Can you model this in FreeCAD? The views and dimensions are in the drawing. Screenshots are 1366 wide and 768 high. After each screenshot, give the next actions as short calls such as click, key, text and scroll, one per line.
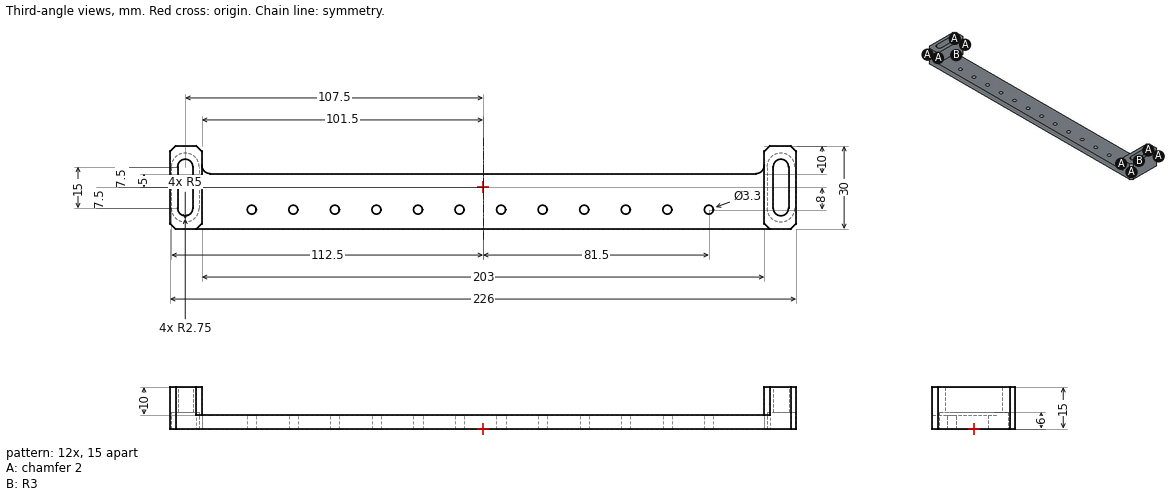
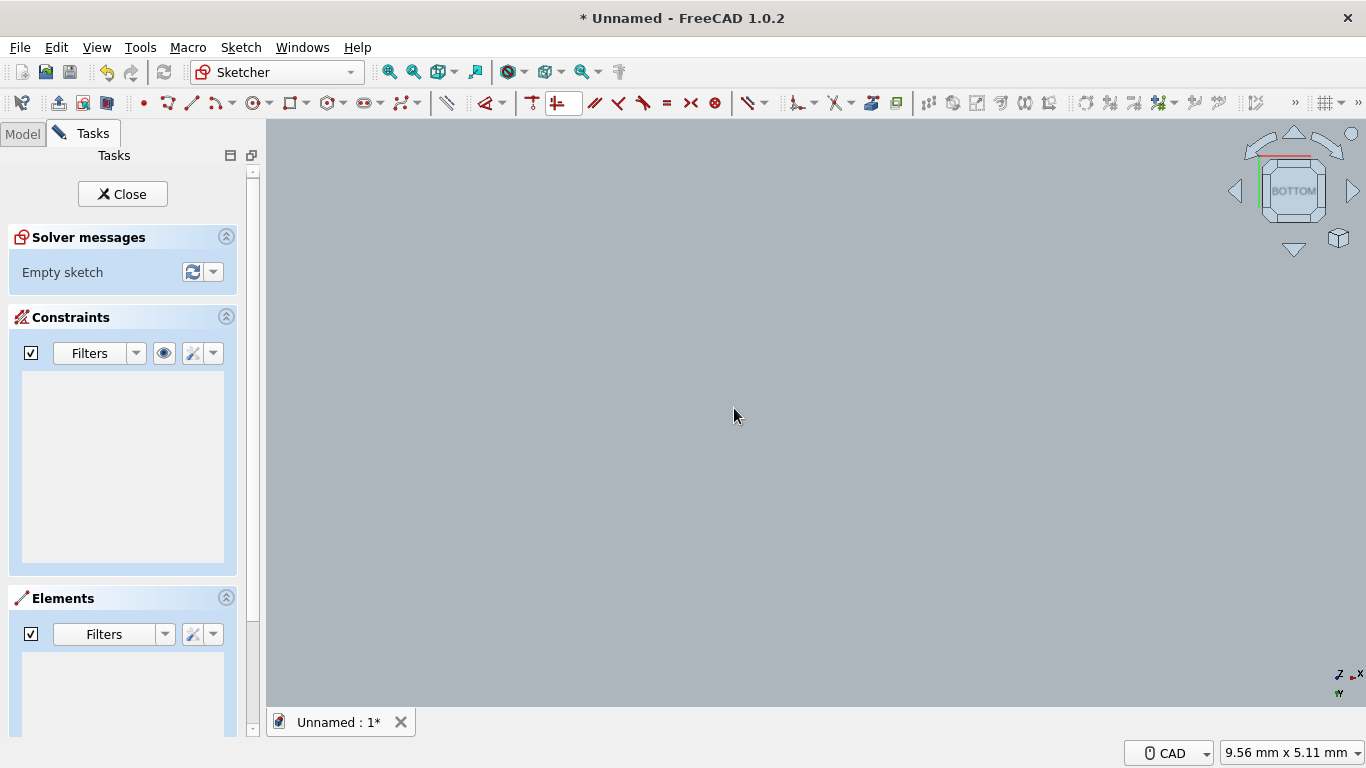
click(254, 104)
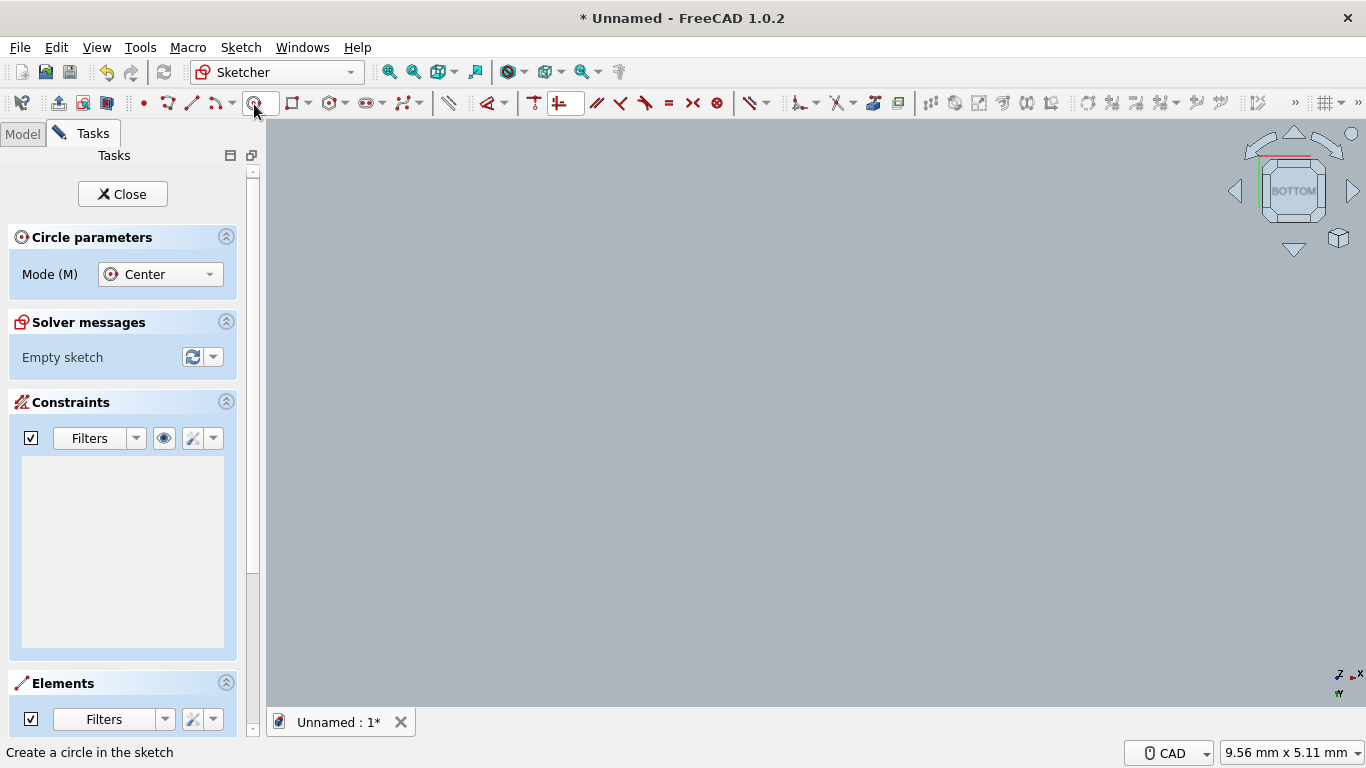
click(747, 413)
move(882, 279)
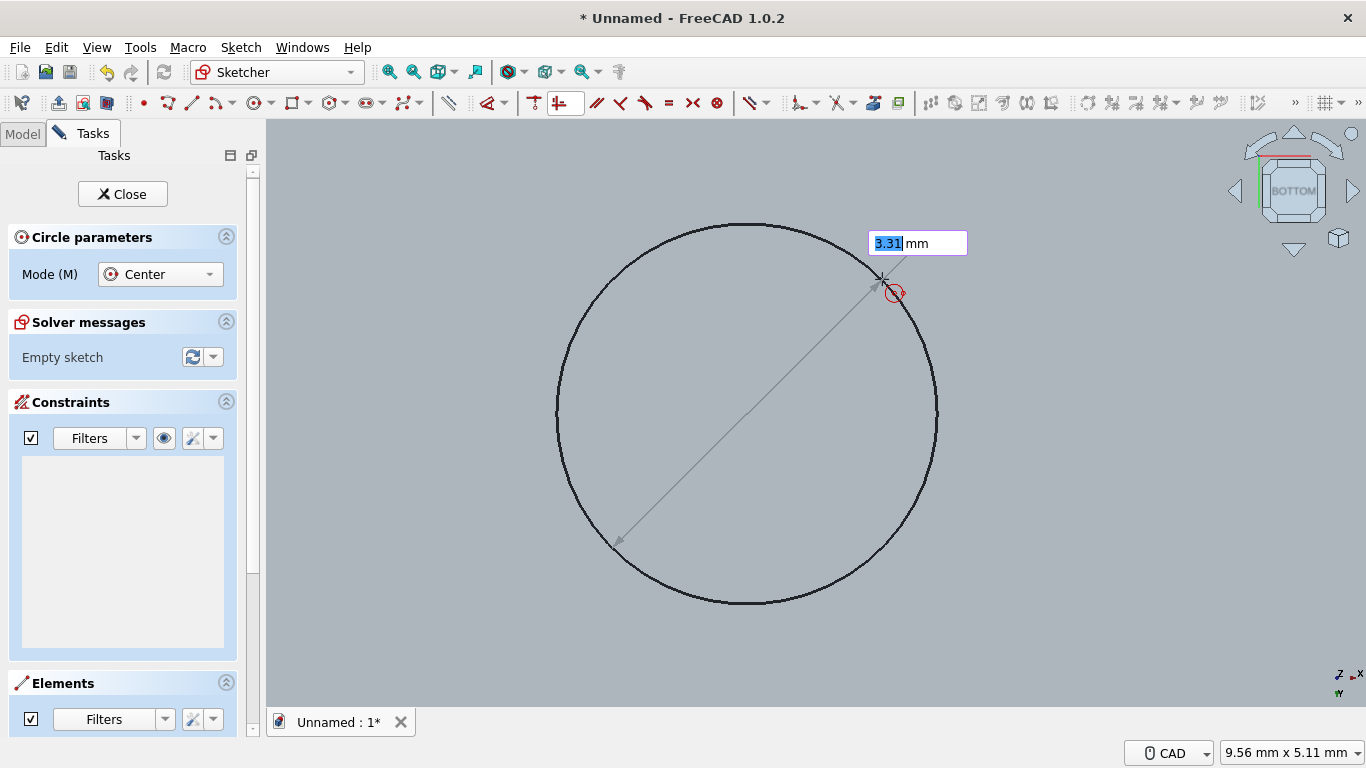
text(3.3)
key(Return)
key(Escape)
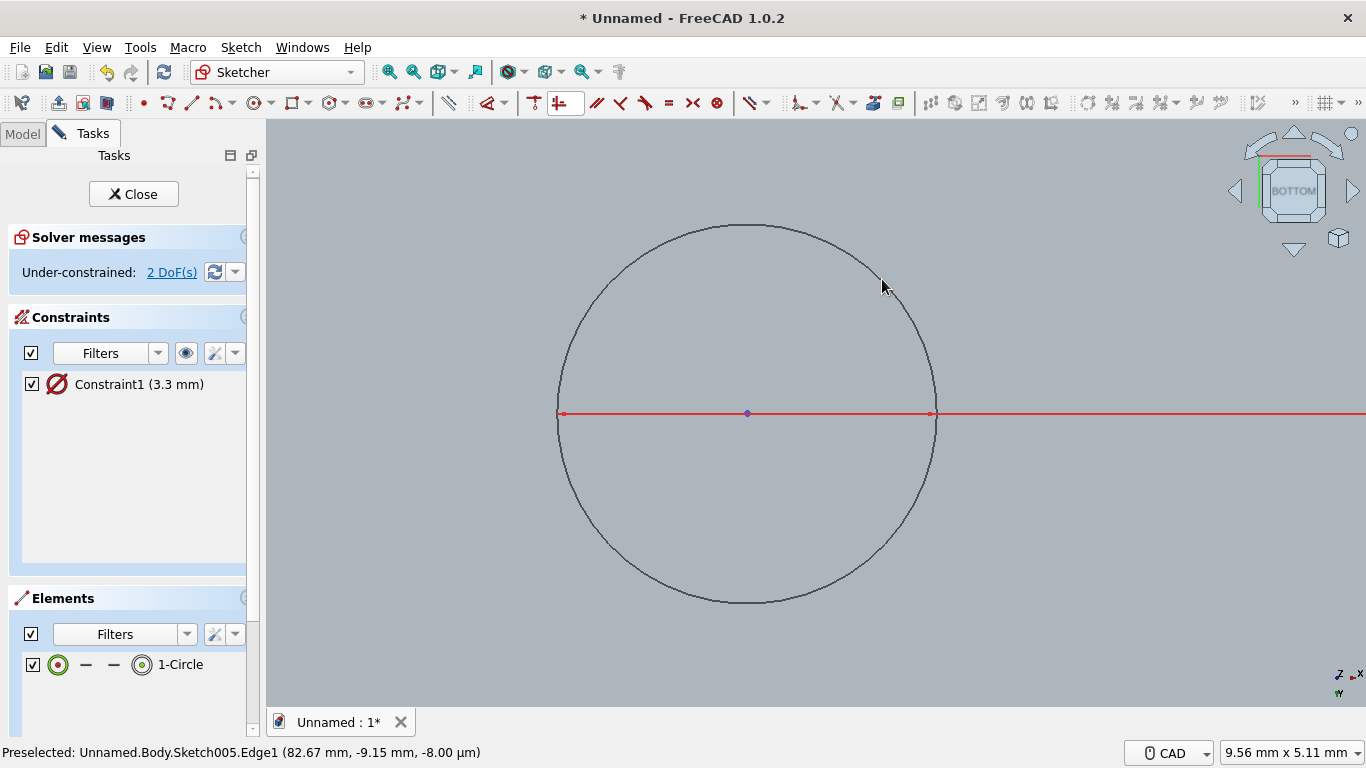
key(d)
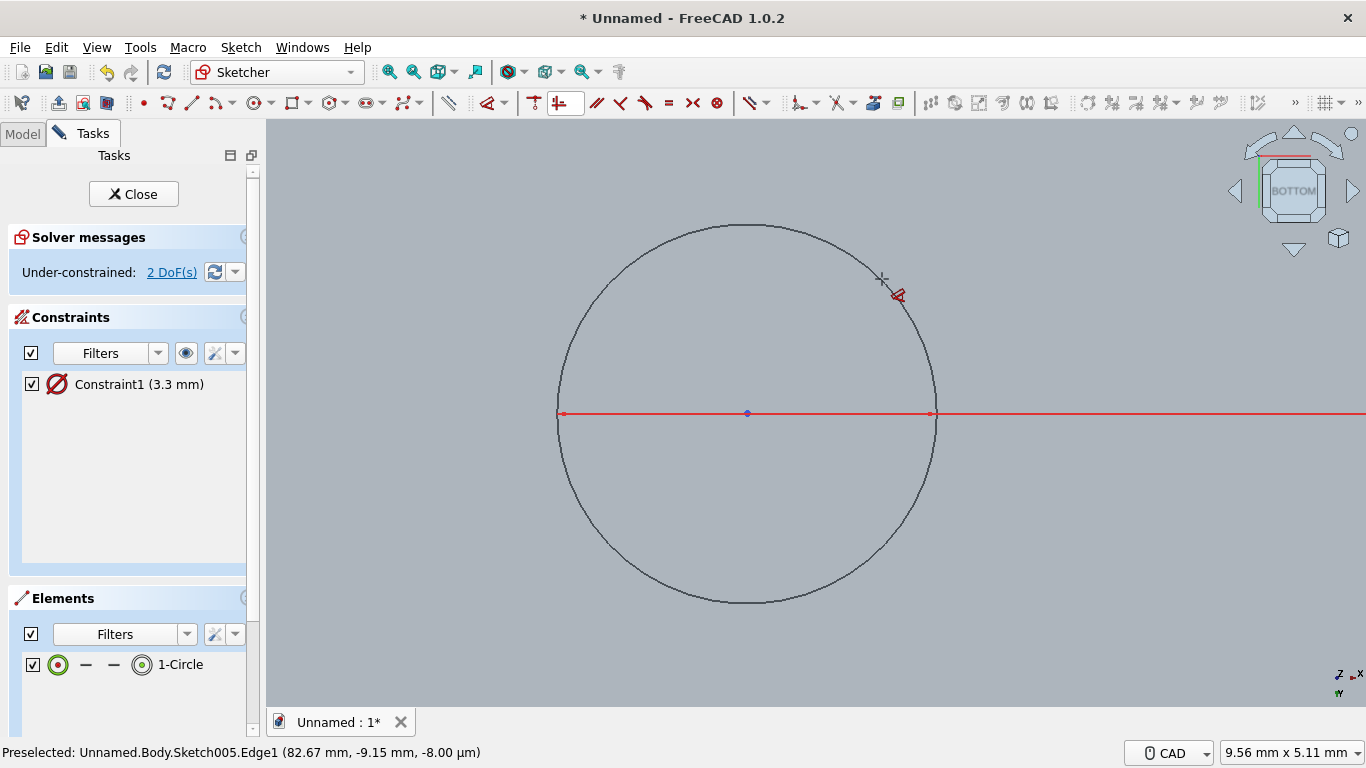
click(747, 414)
click(781, 547)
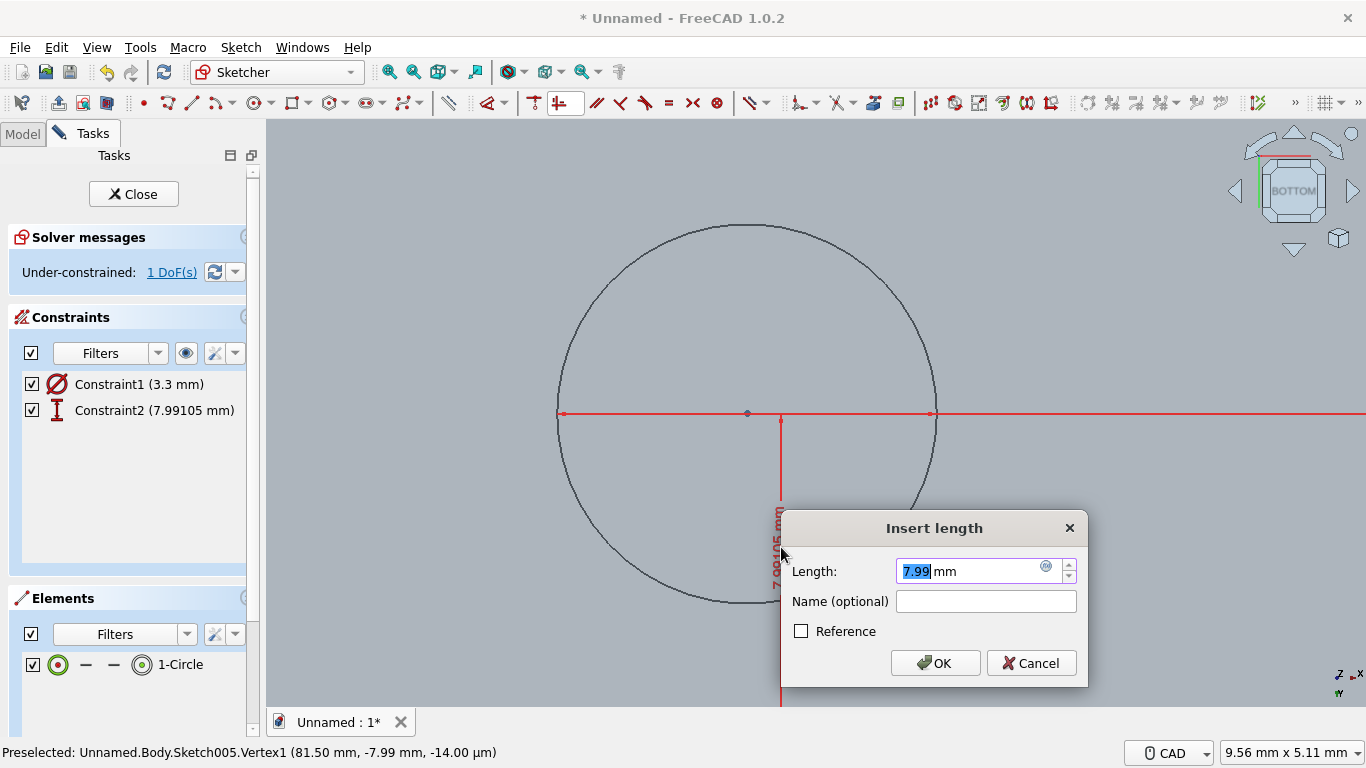
text(8)
key(Return)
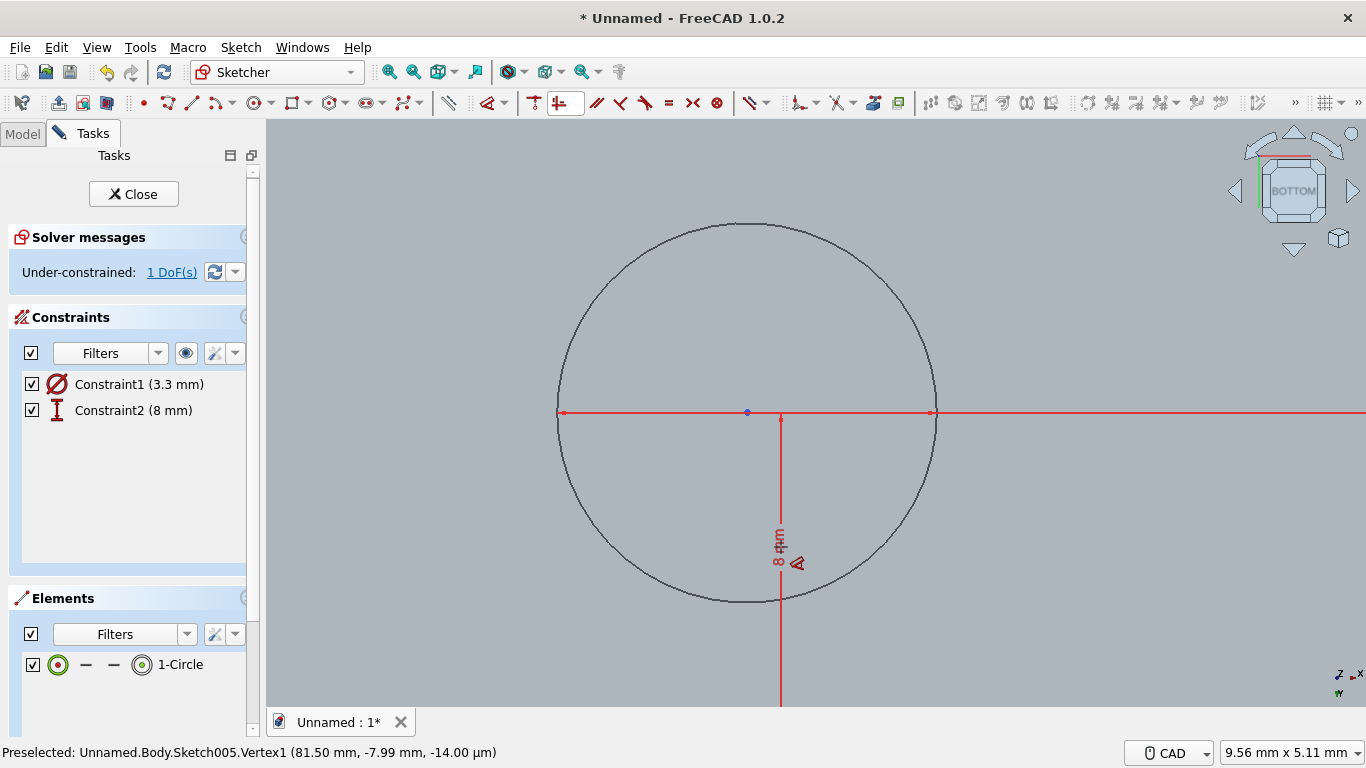
click(747, 413)
click(521, 379)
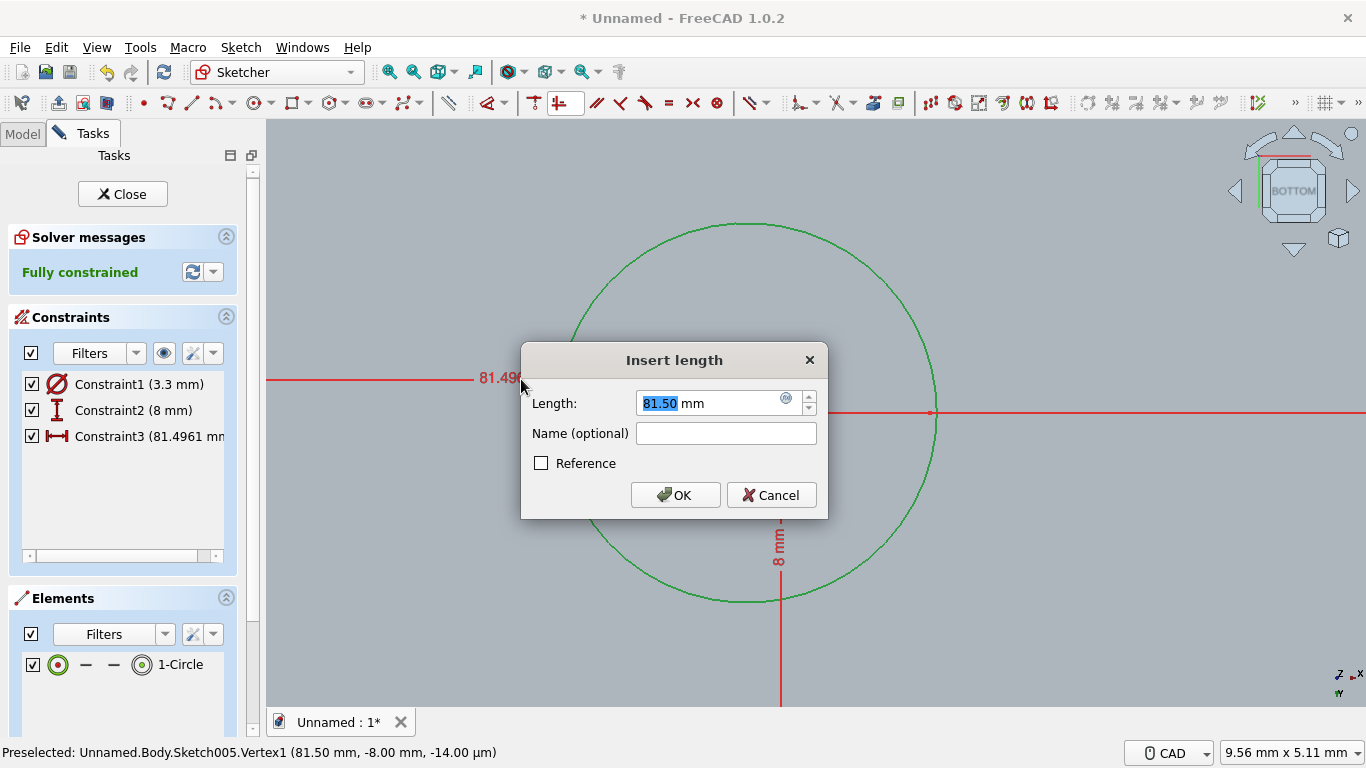
text(81.5)
key(Return)
key(Escape)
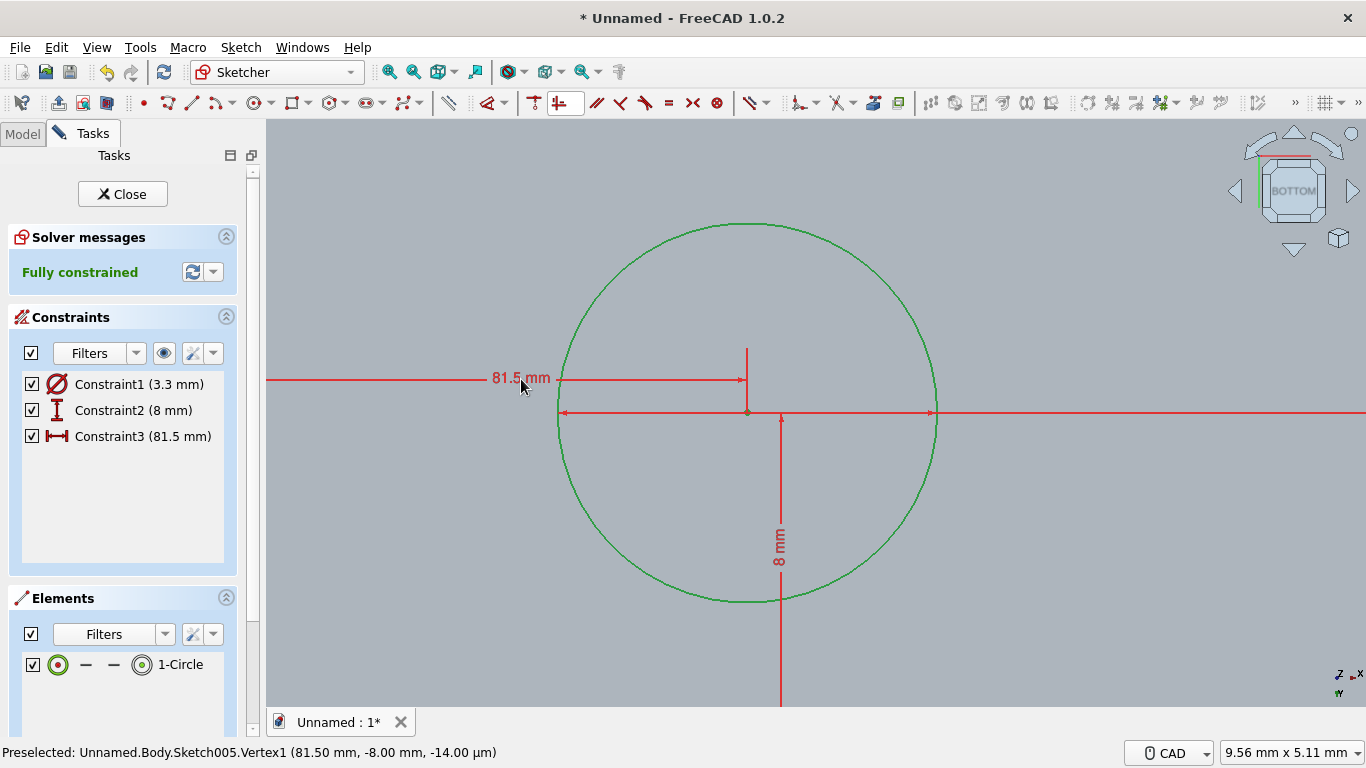
click(123, 194)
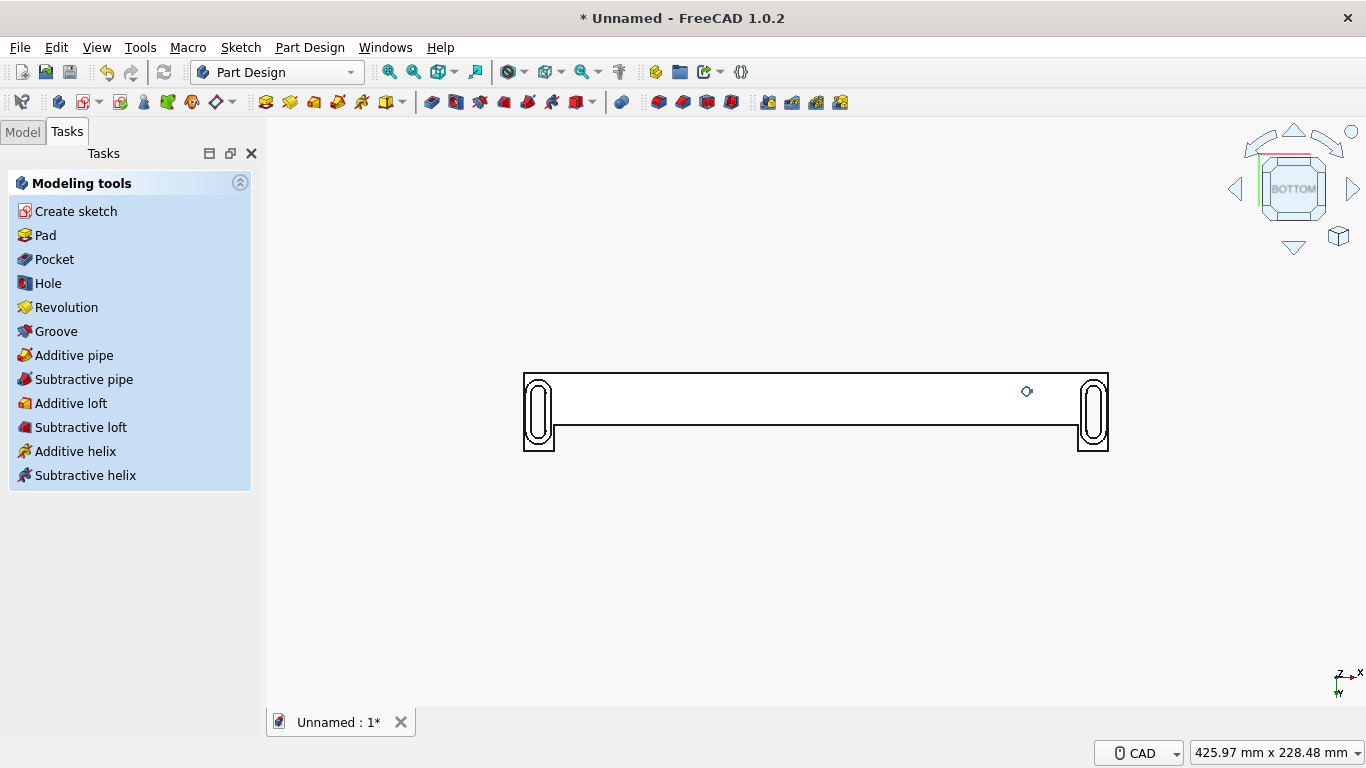
click(432, 102)